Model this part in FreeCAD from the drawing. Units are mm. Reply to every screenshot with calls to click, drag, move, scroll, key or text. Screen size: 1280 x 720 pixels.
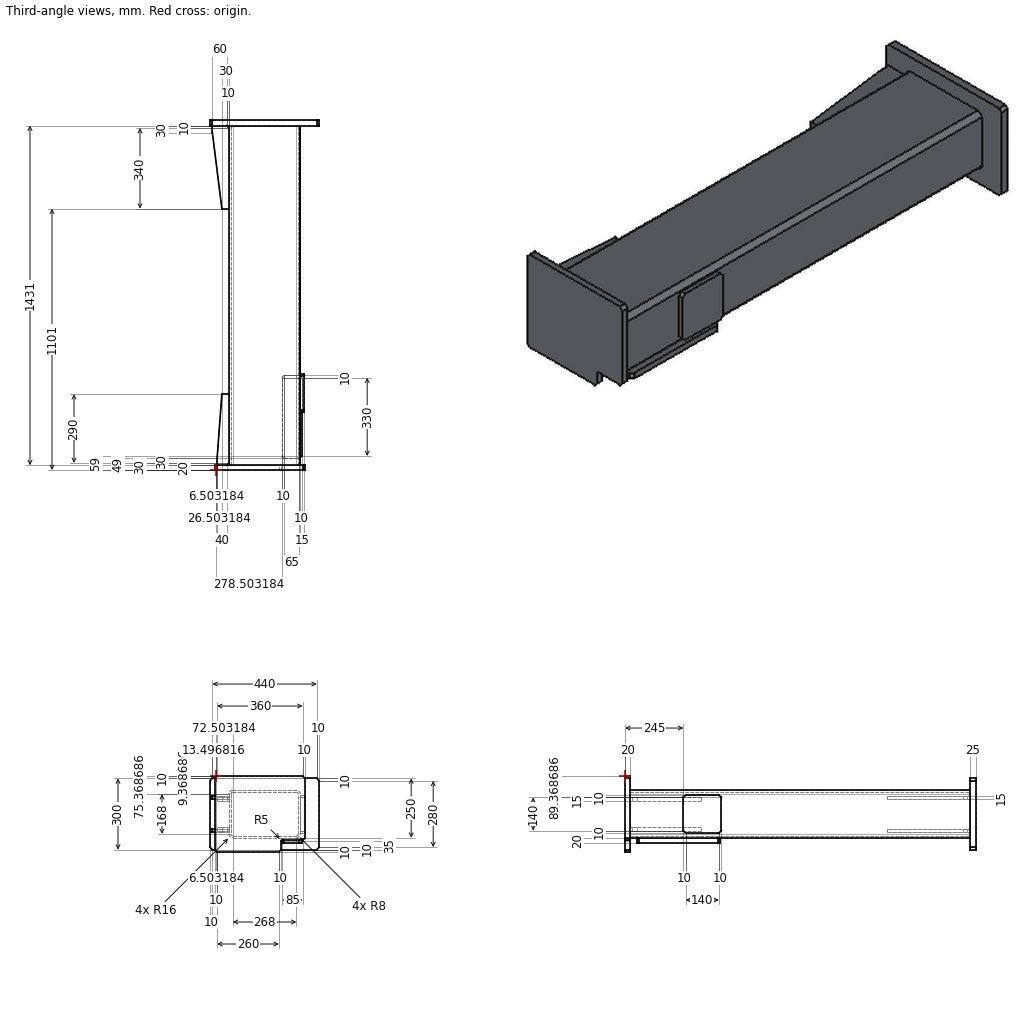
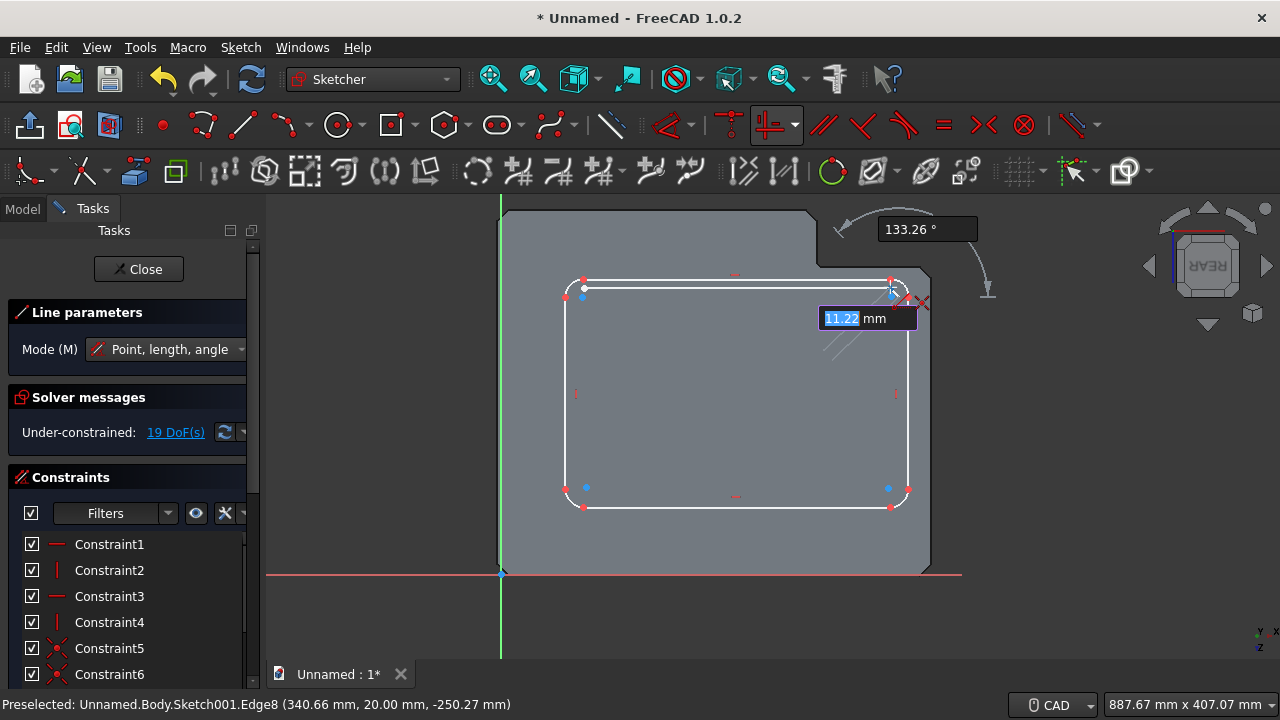
scroll(899, 489, up, 3)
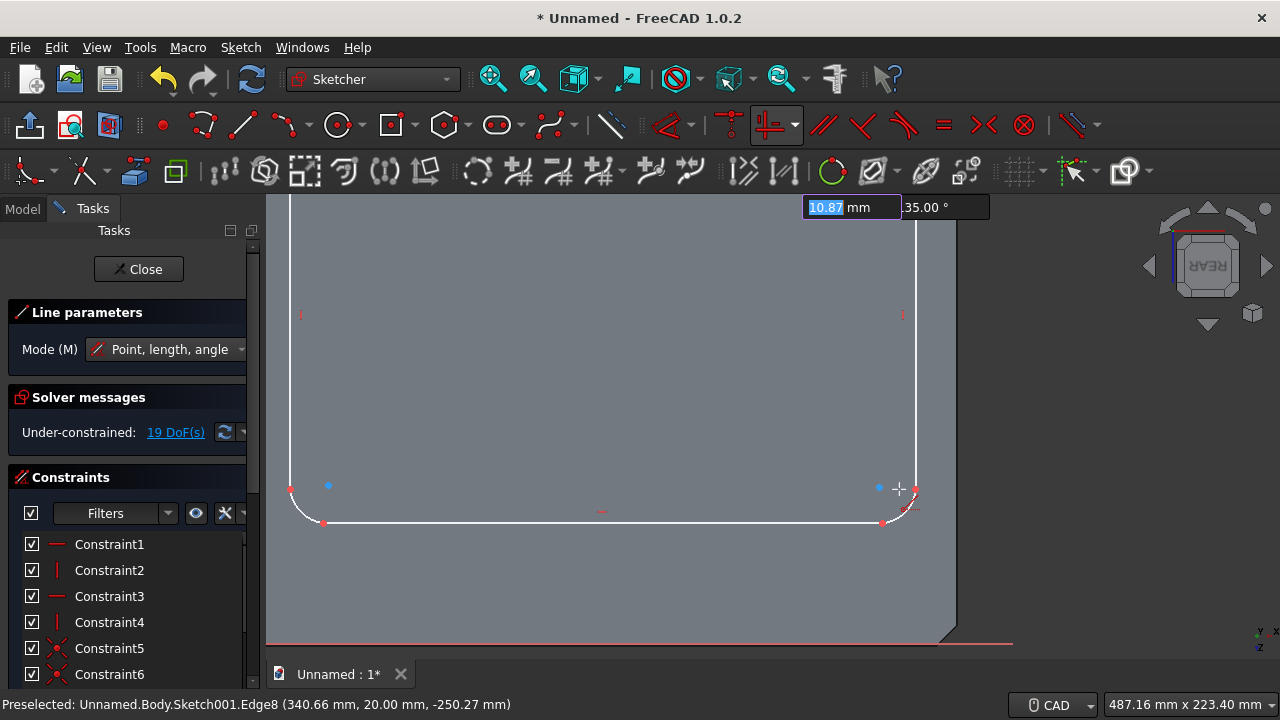
click(899, 488)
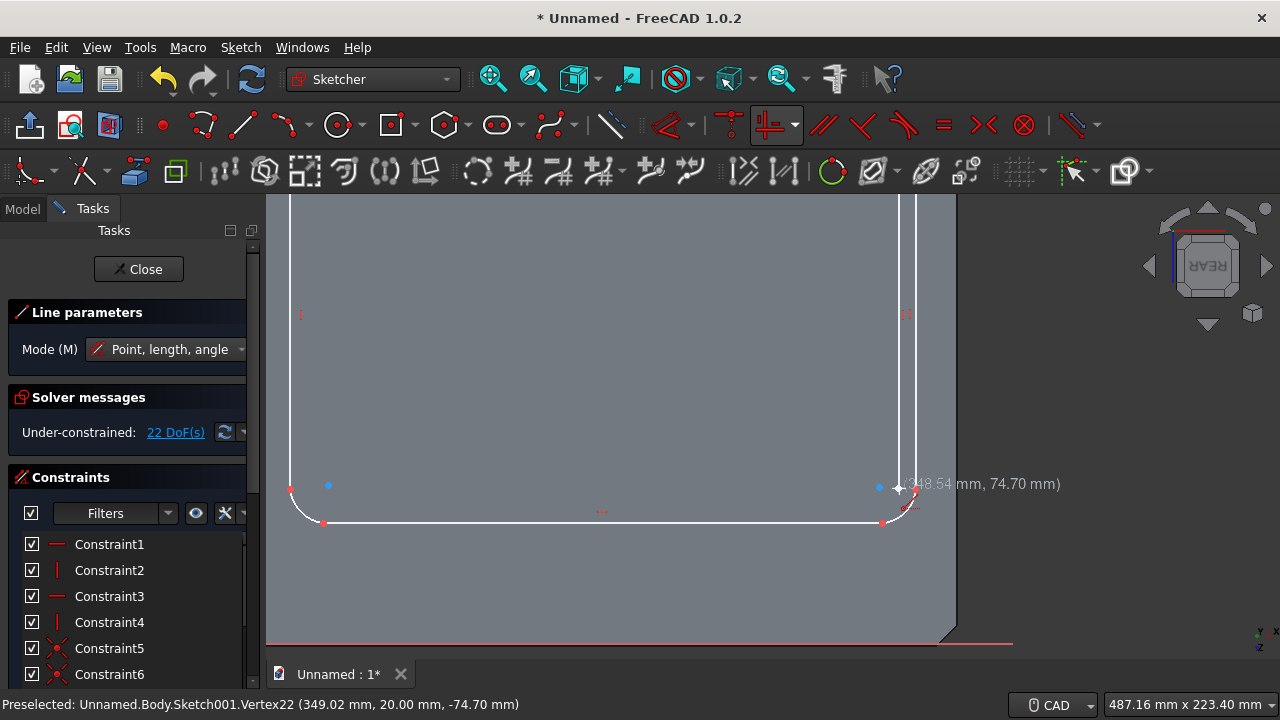
click(882, 504)
click(324, 504)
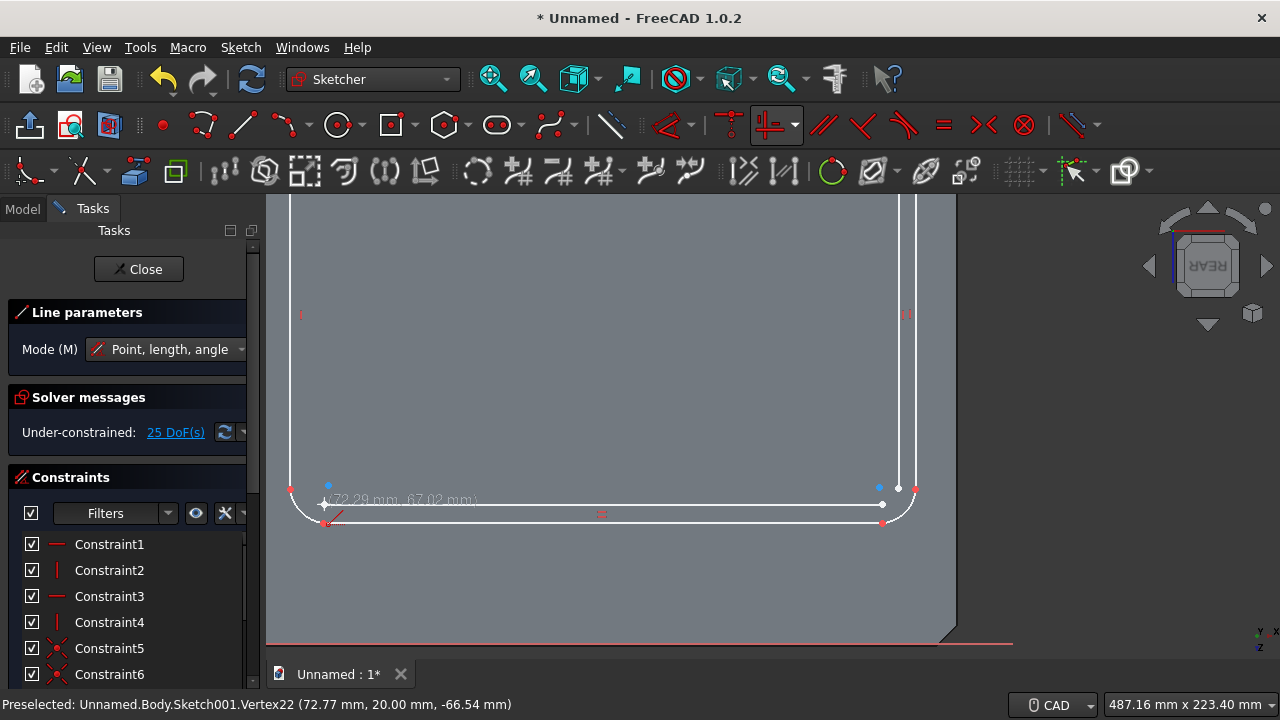
click(308, 488)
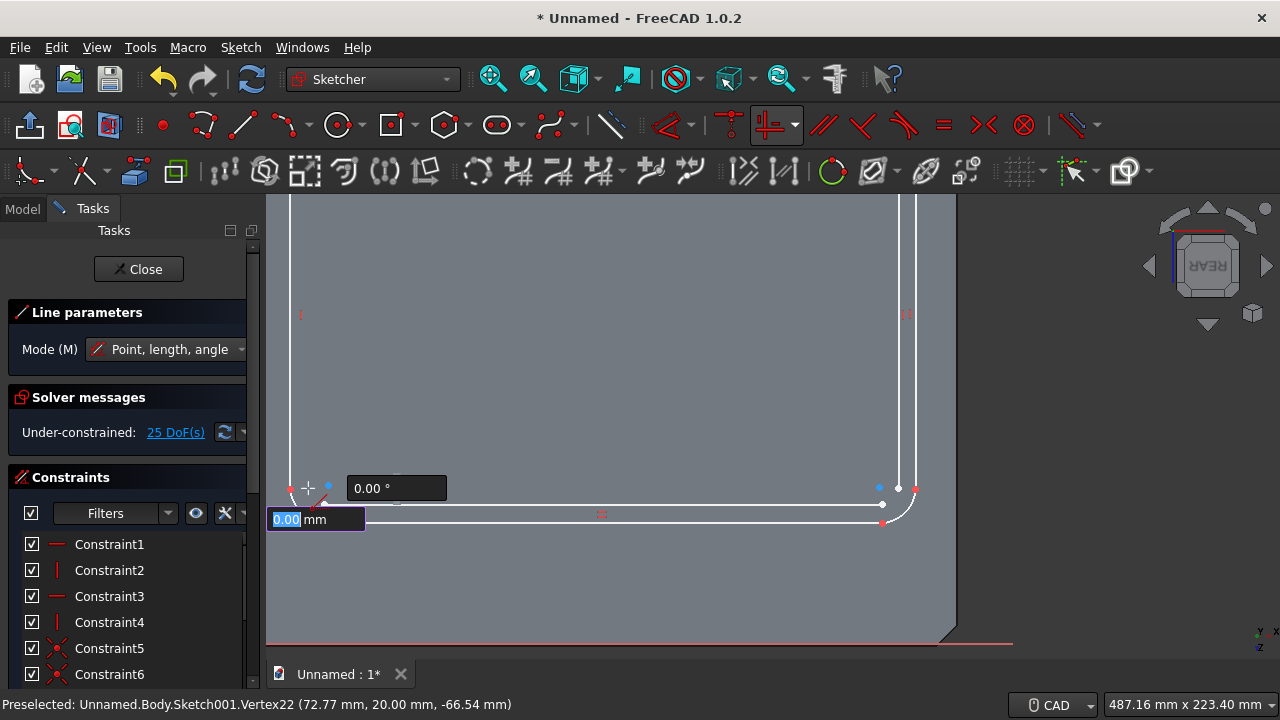
scroll(899, 490, down, 3)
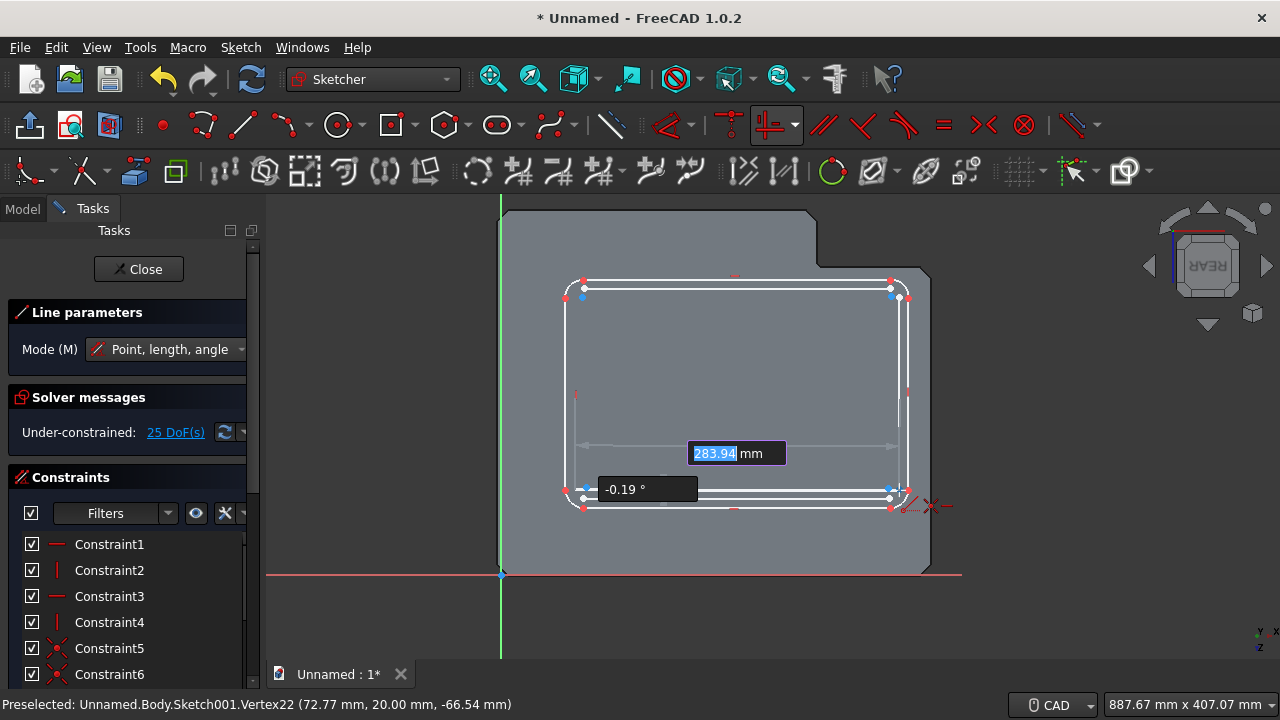
scroll(575, 297, up, 3)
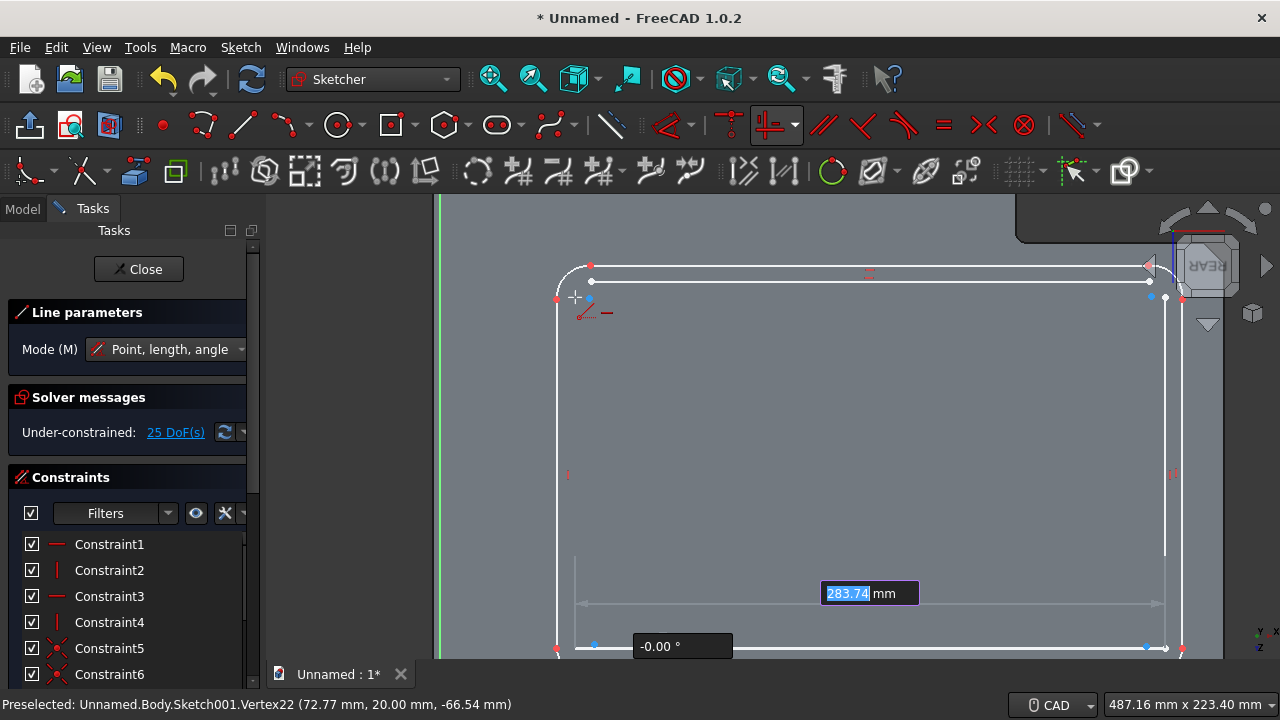
click(575, 297)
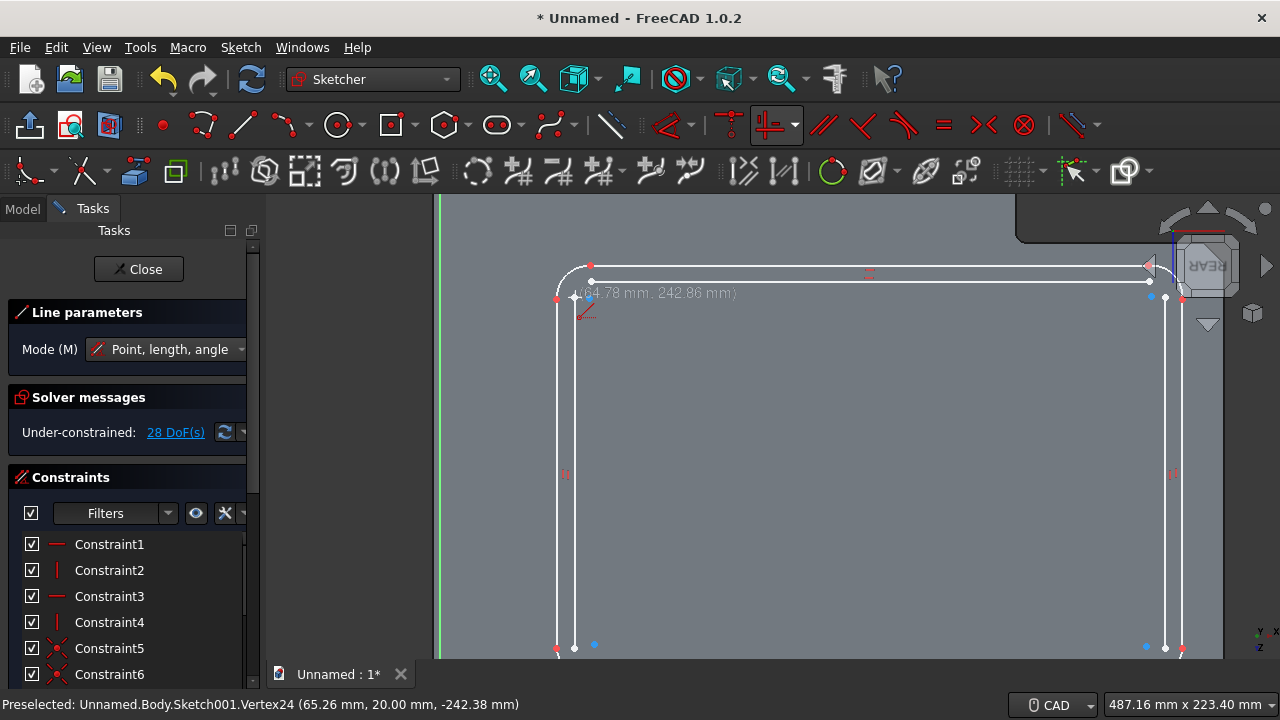
key(g)
key(3)
key(a)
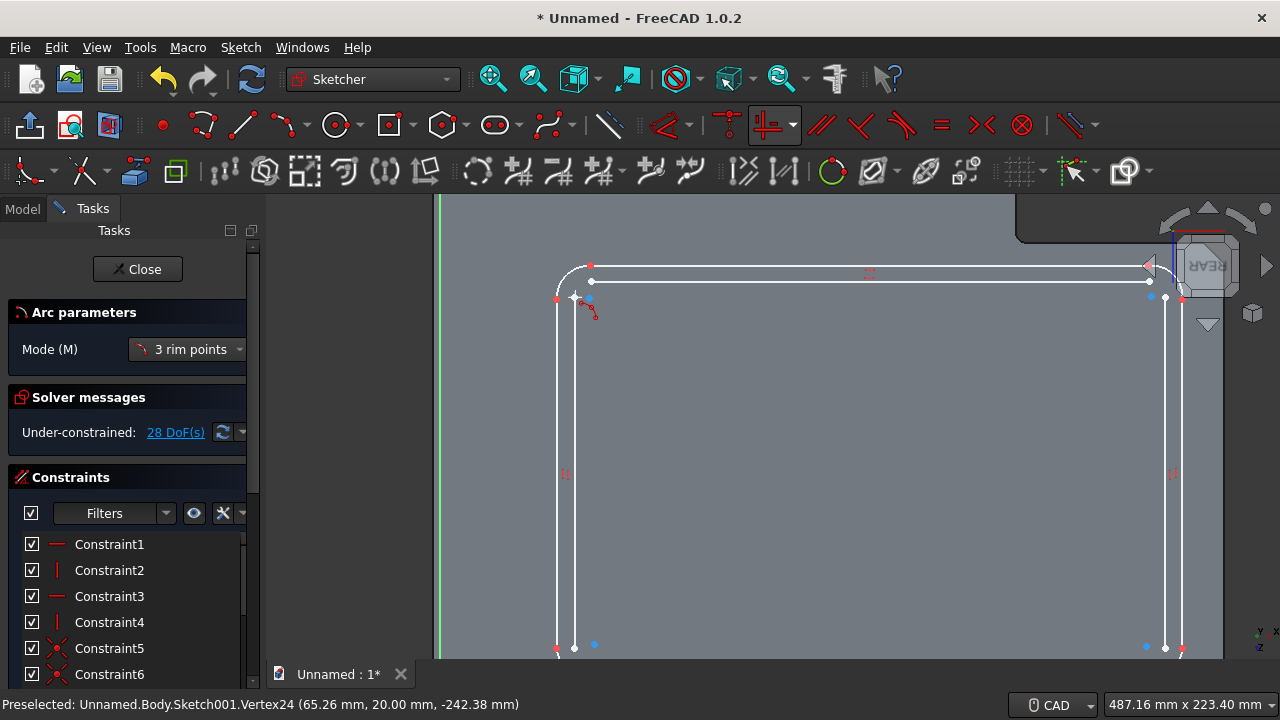
scroll(575, 296, down, 3)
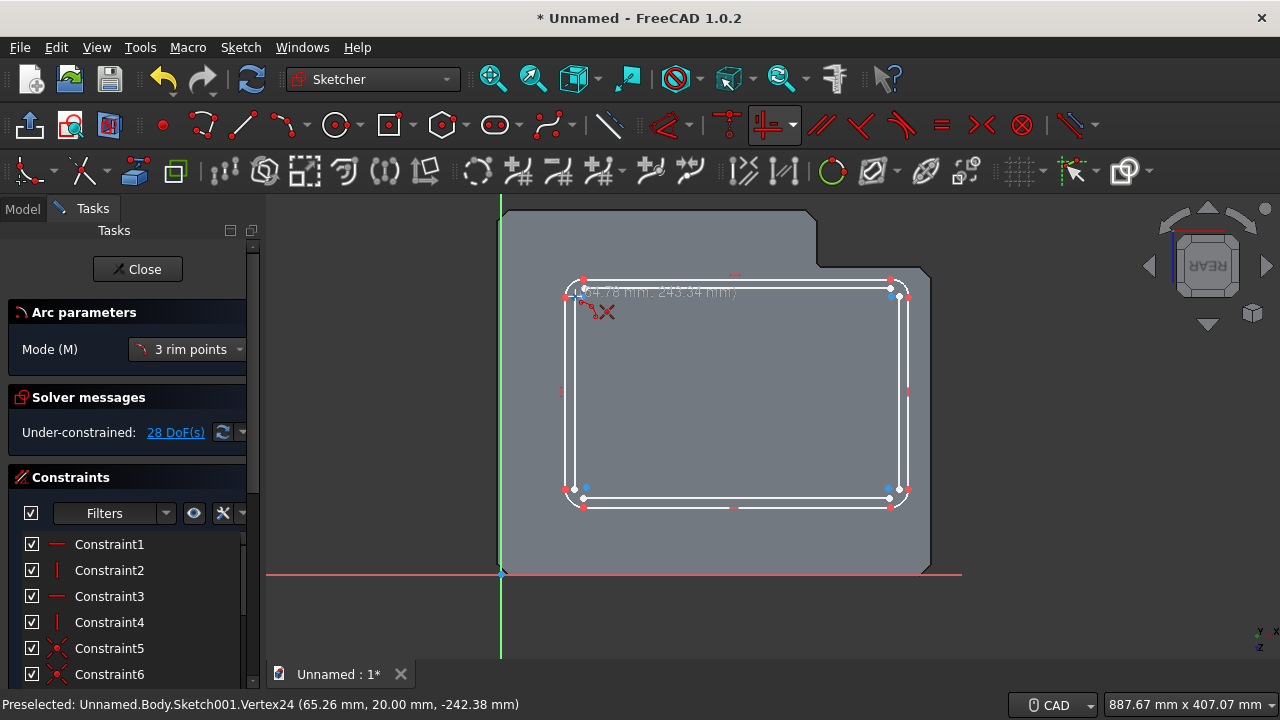
scroll(890, 287, up, 3)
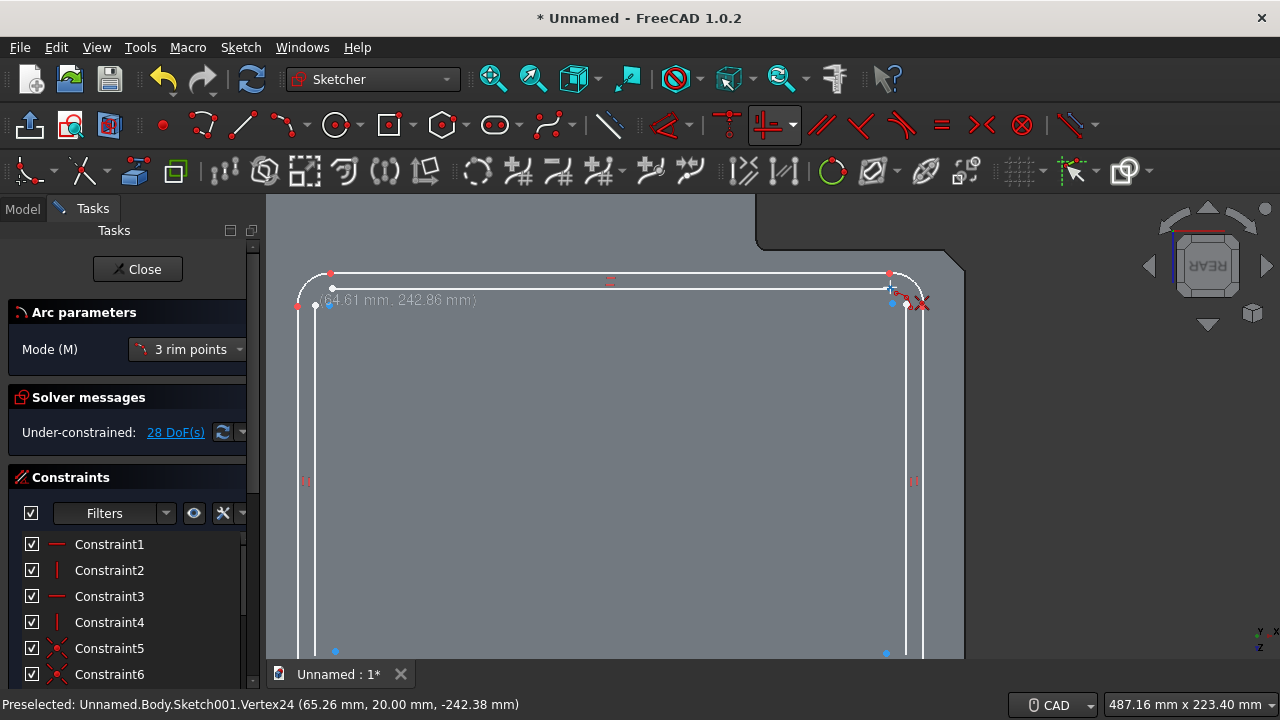
click(890, 289)
click(906, 305)